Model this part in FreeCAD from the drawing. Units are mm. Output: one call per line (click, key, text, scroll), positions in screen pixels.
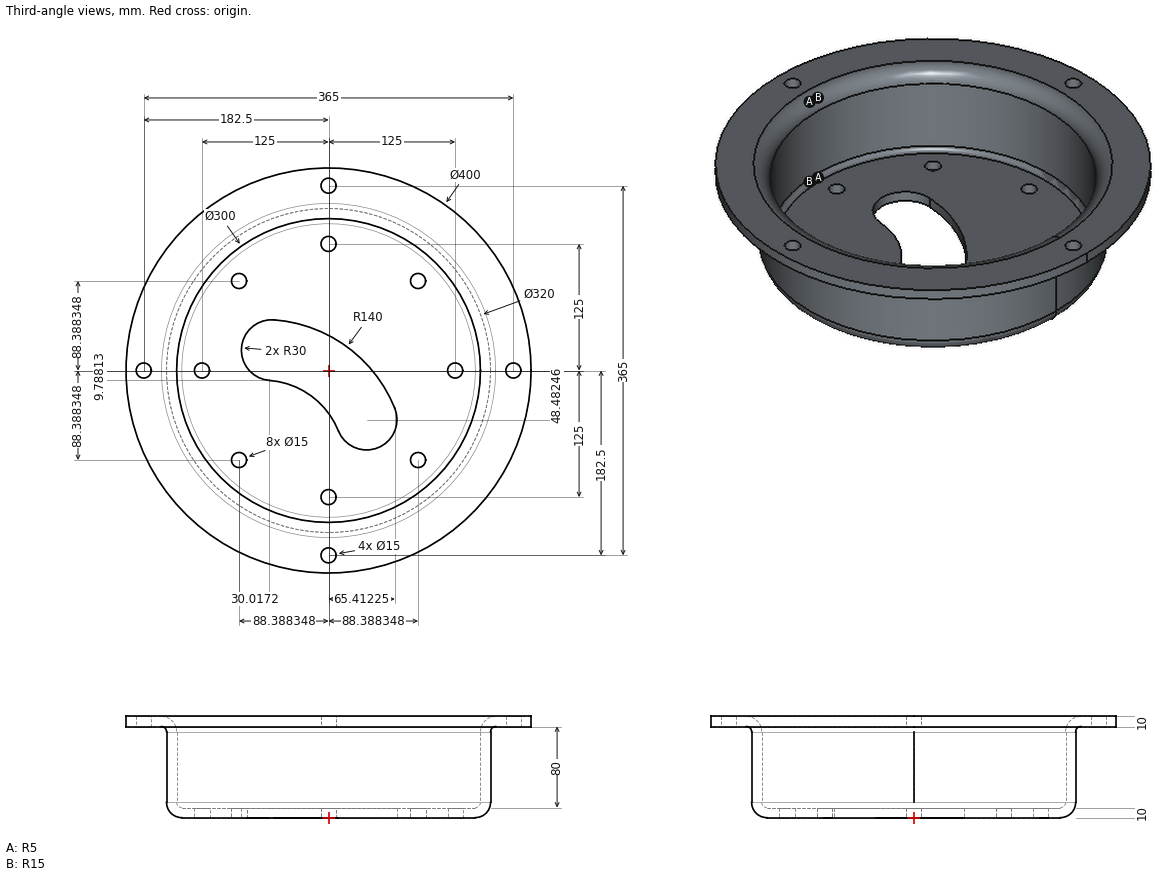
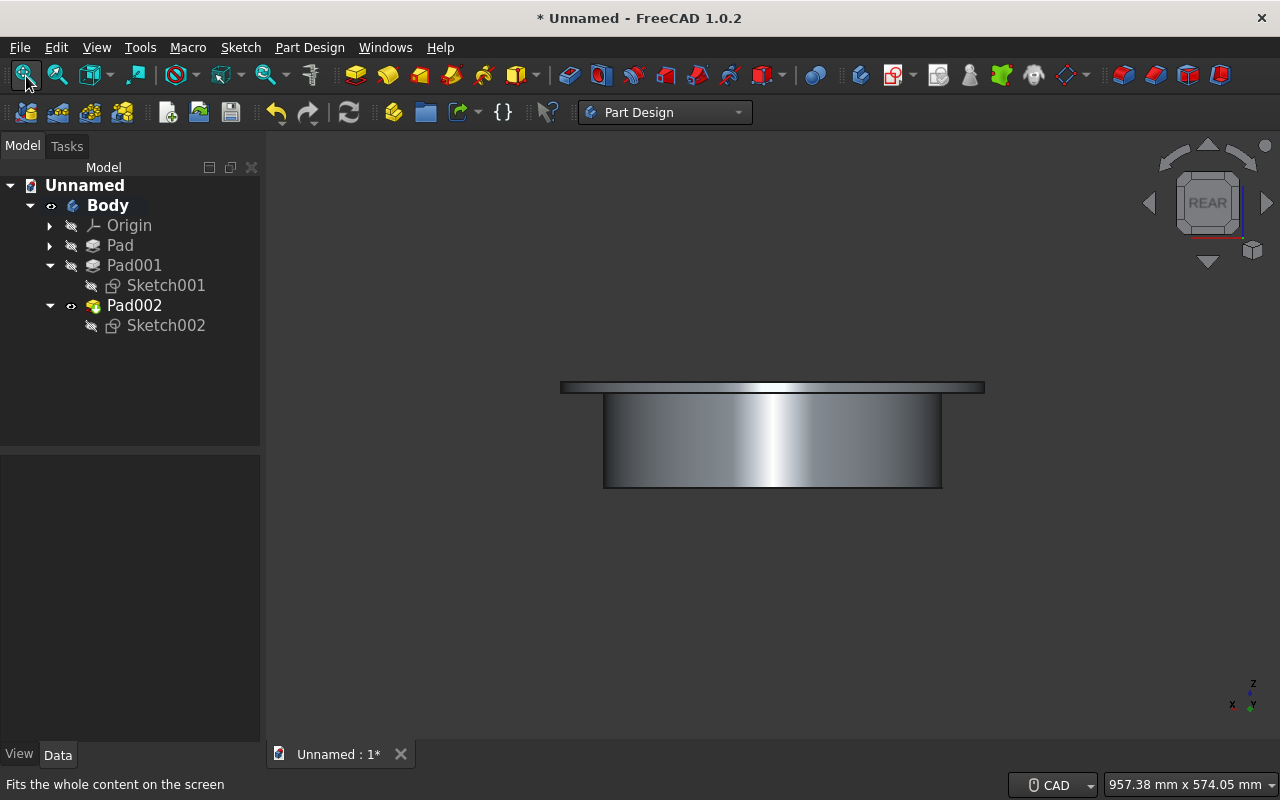
click(26, 76)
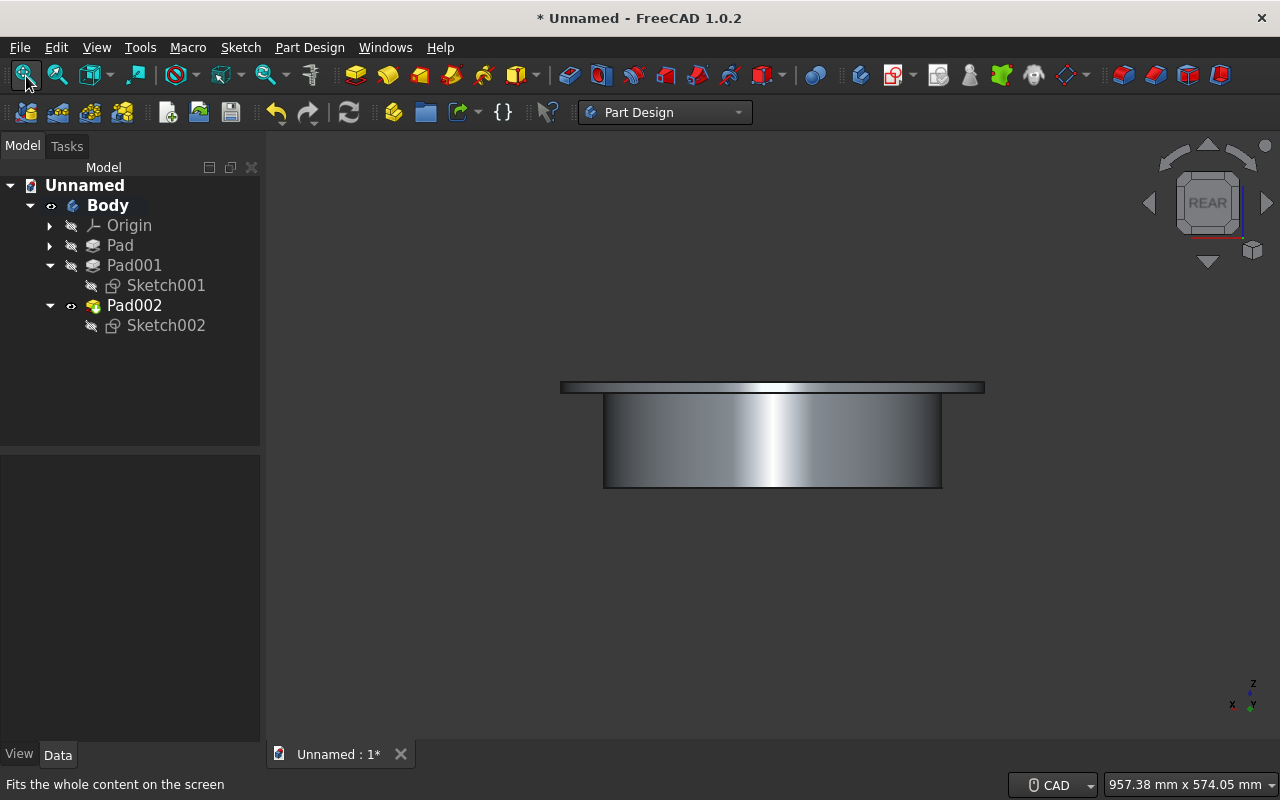
key(6)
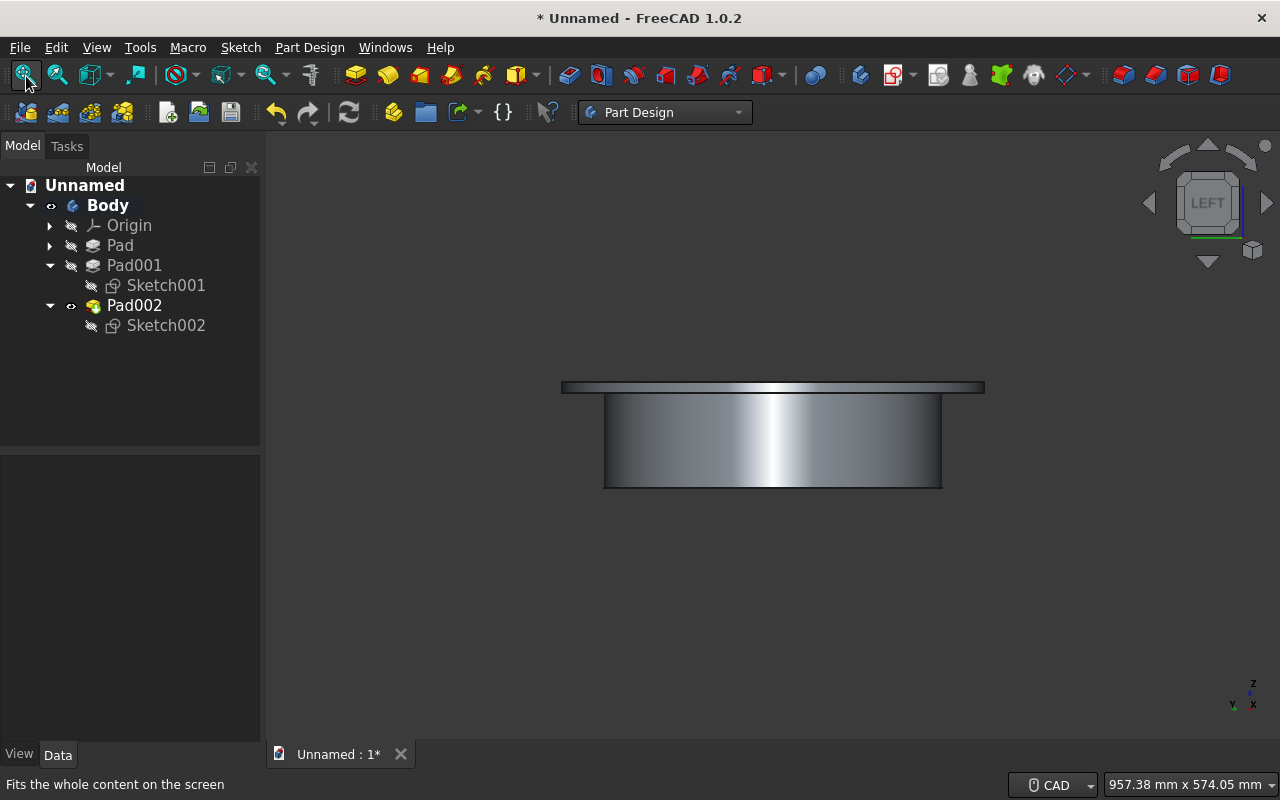
click(26, 76)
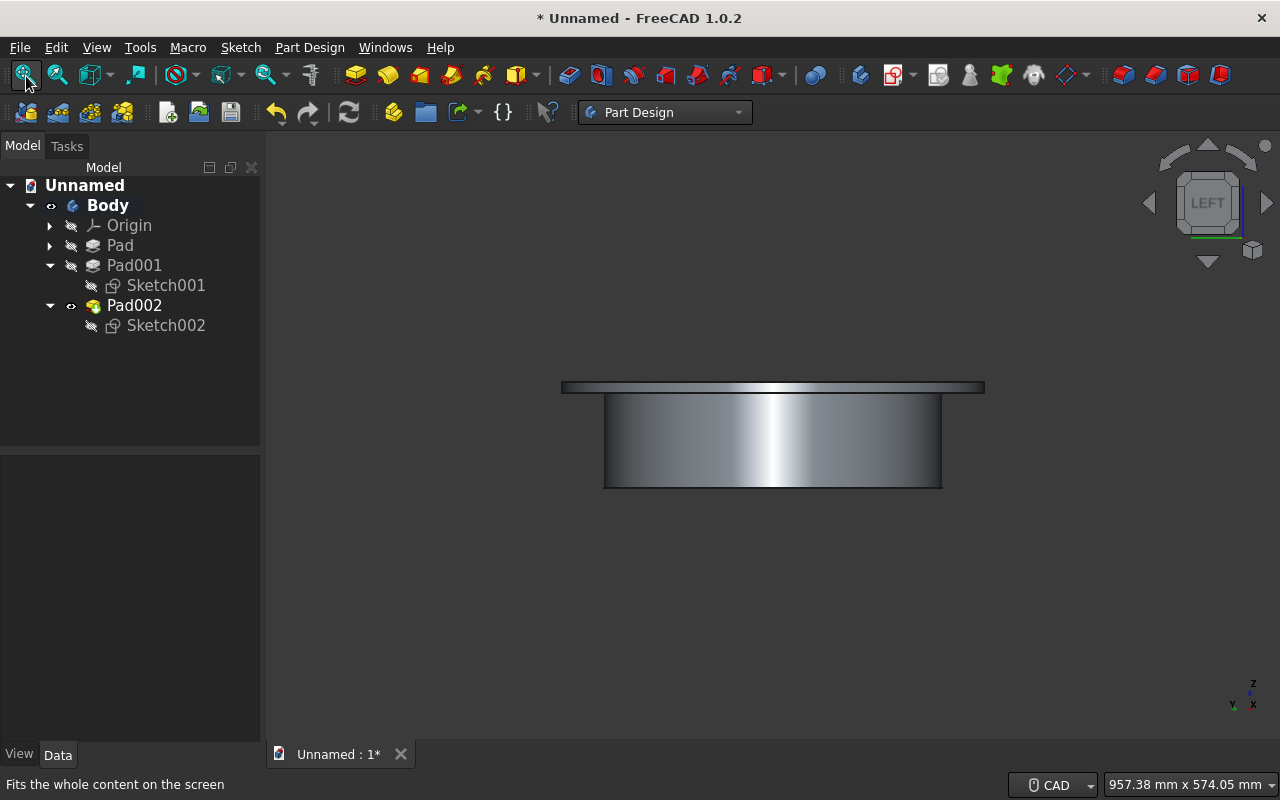
key(v)
key(3)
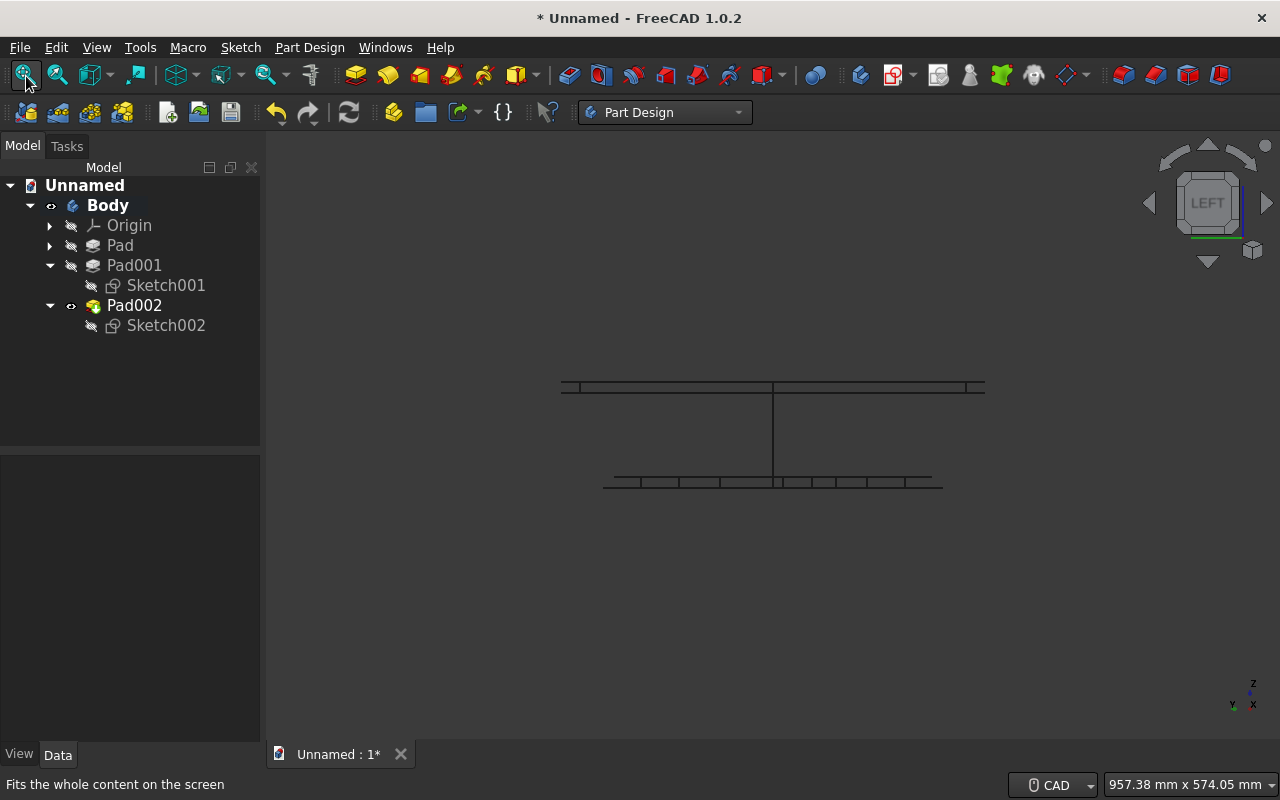
key(0)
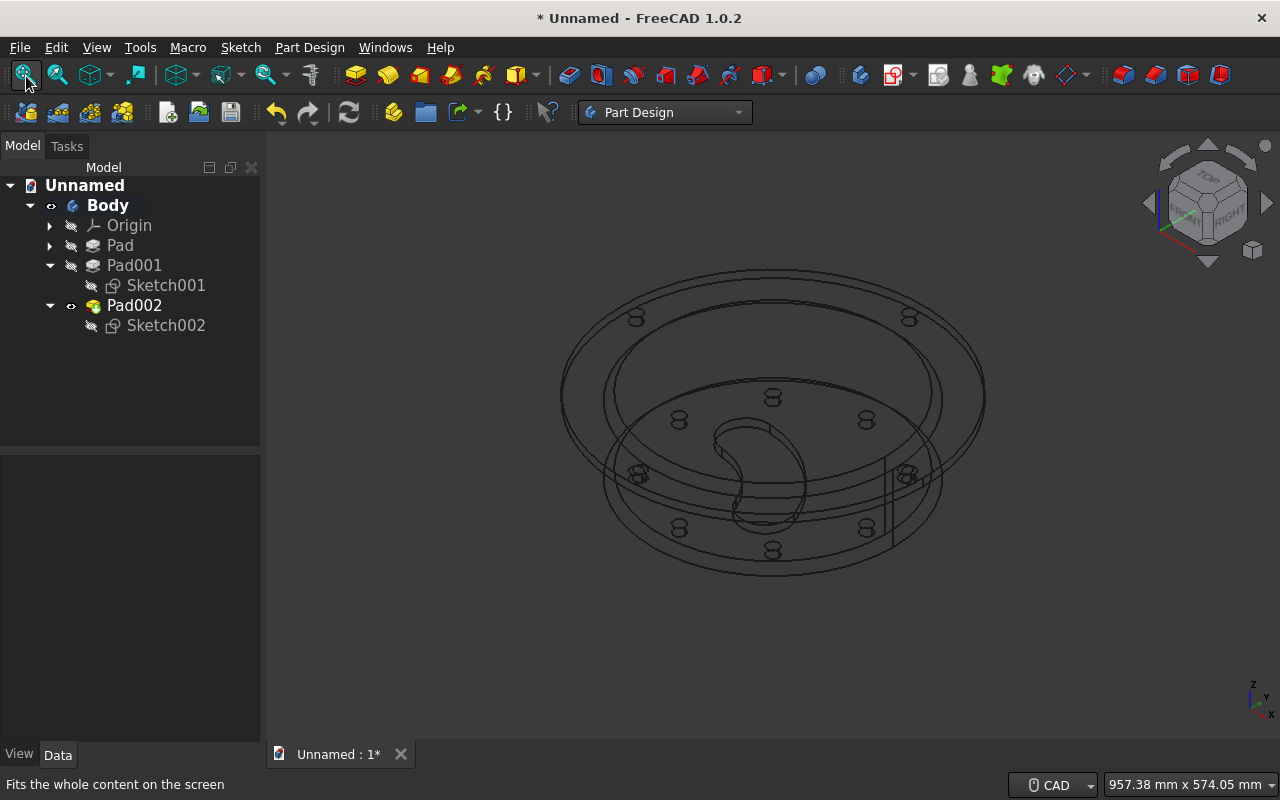
click(661, 404)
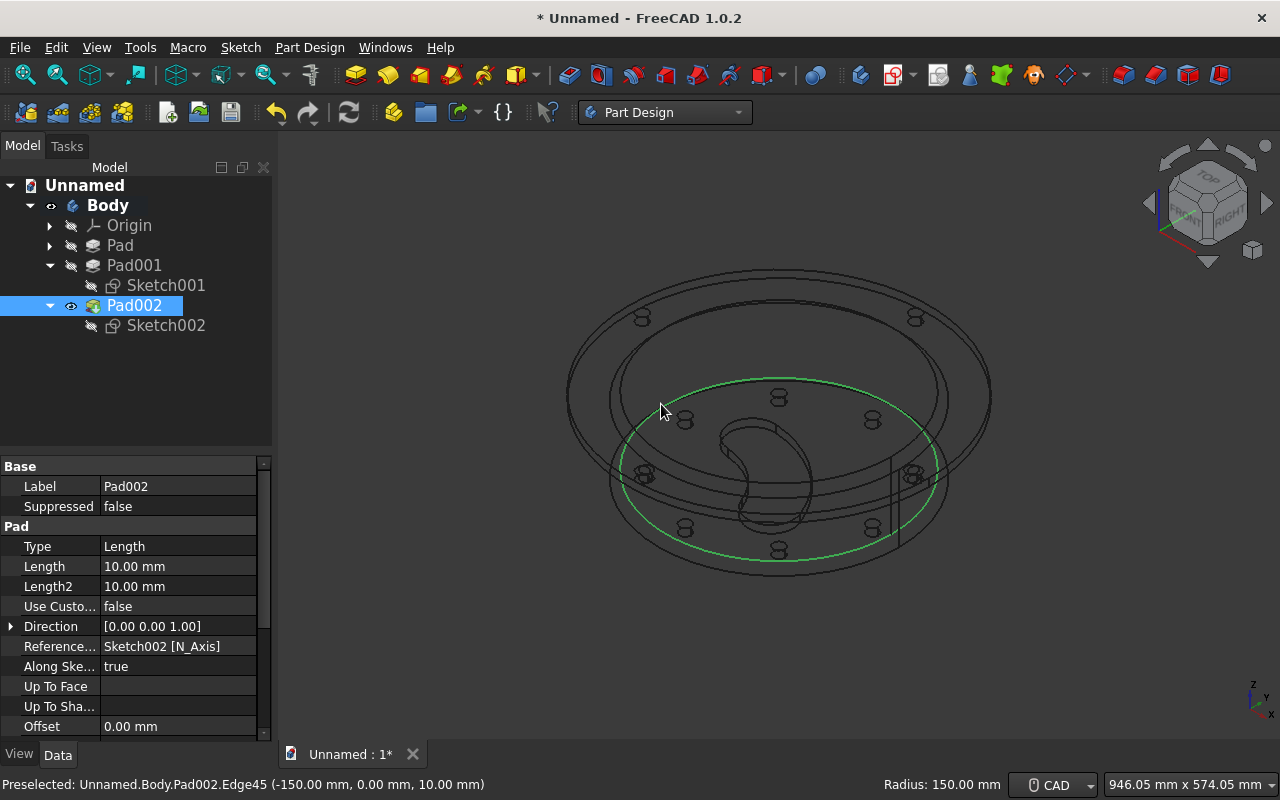
click(612, 384, ctrl)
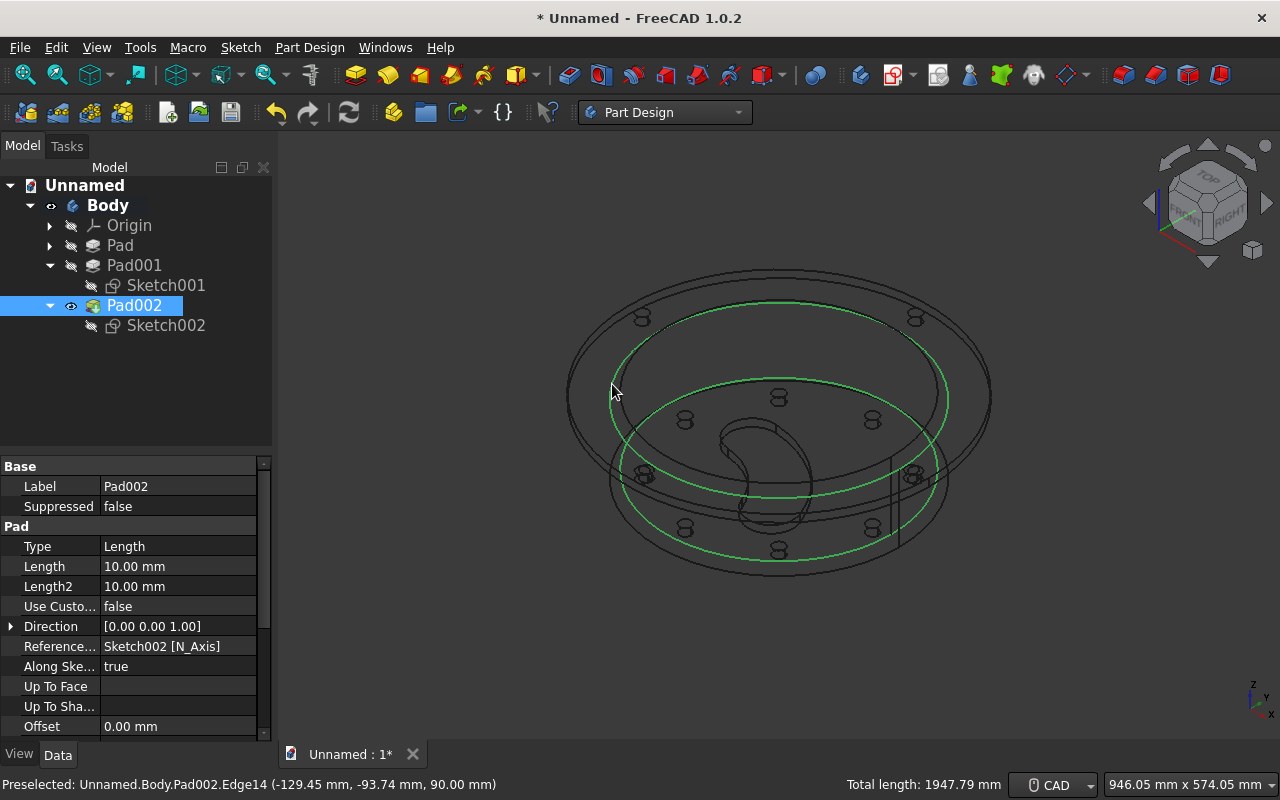
key(v)
key(1)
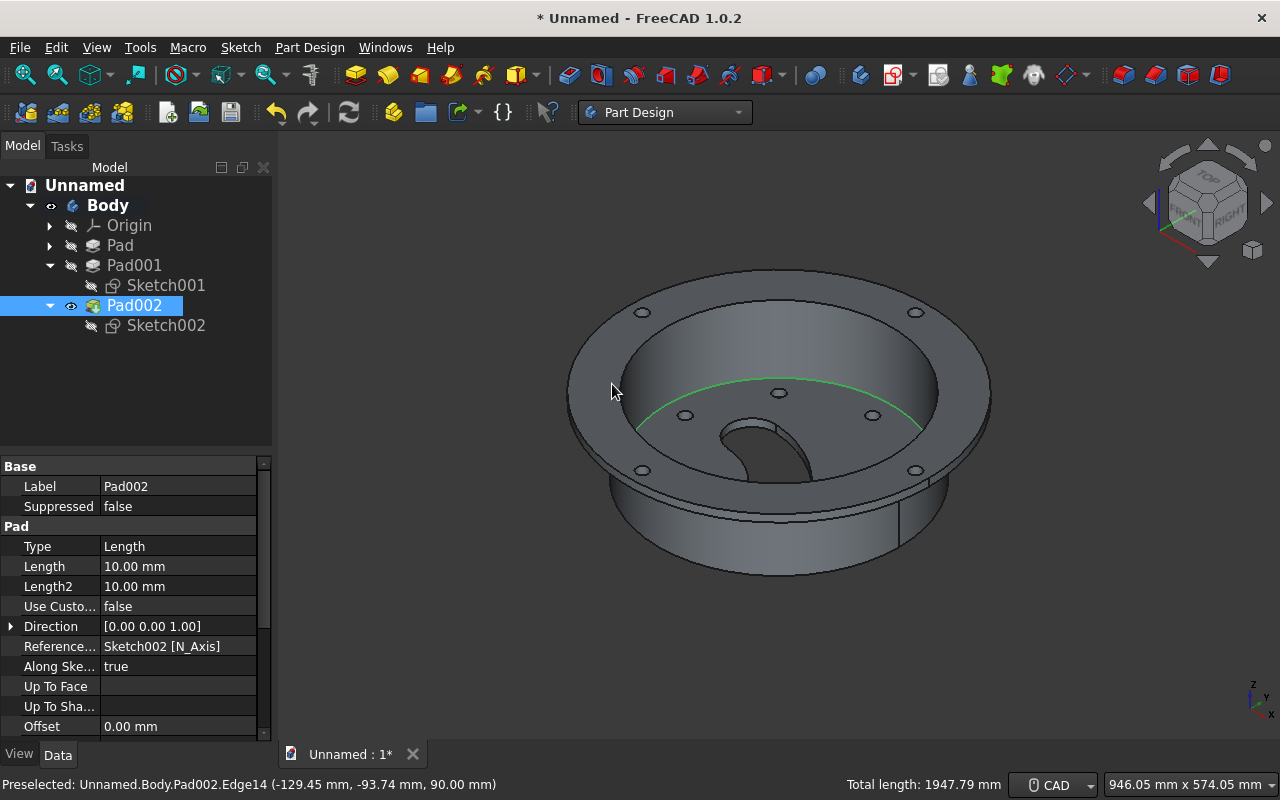
click(1124, 76)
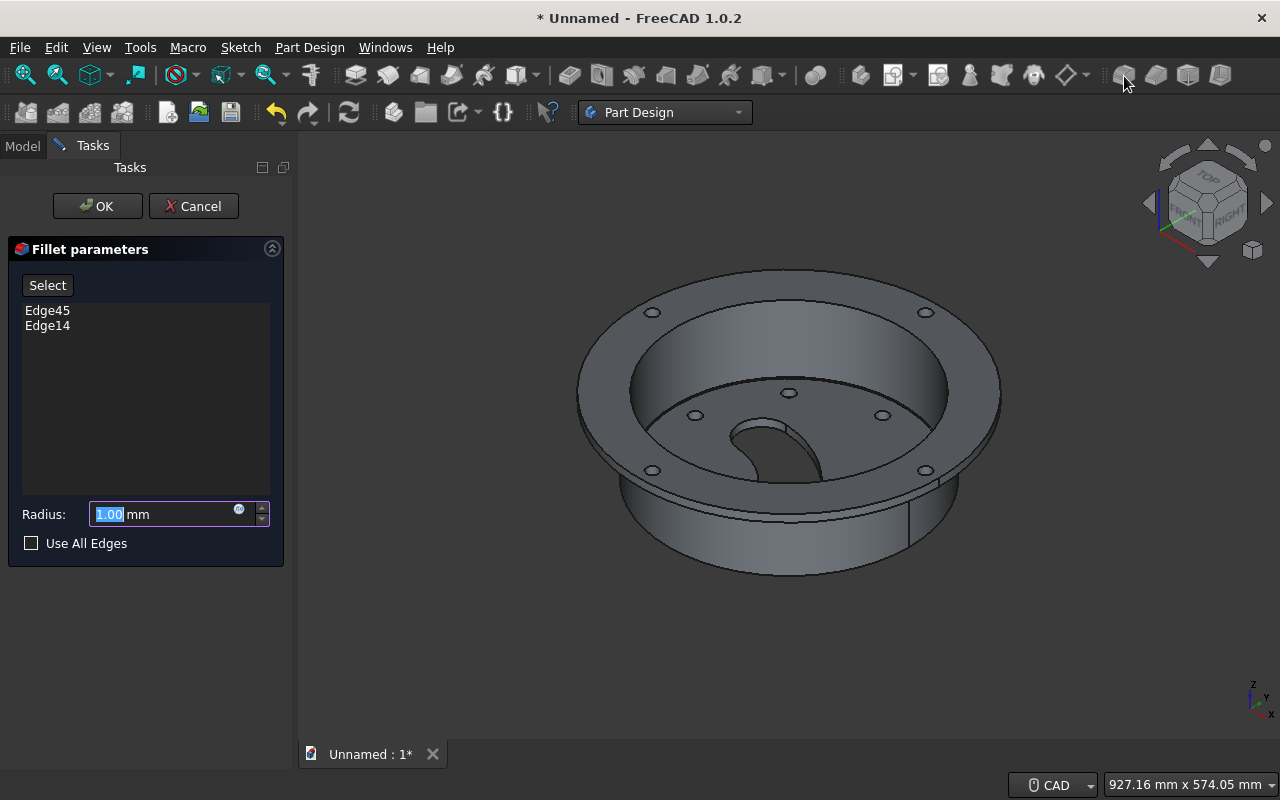
text(5)
key(Tab)